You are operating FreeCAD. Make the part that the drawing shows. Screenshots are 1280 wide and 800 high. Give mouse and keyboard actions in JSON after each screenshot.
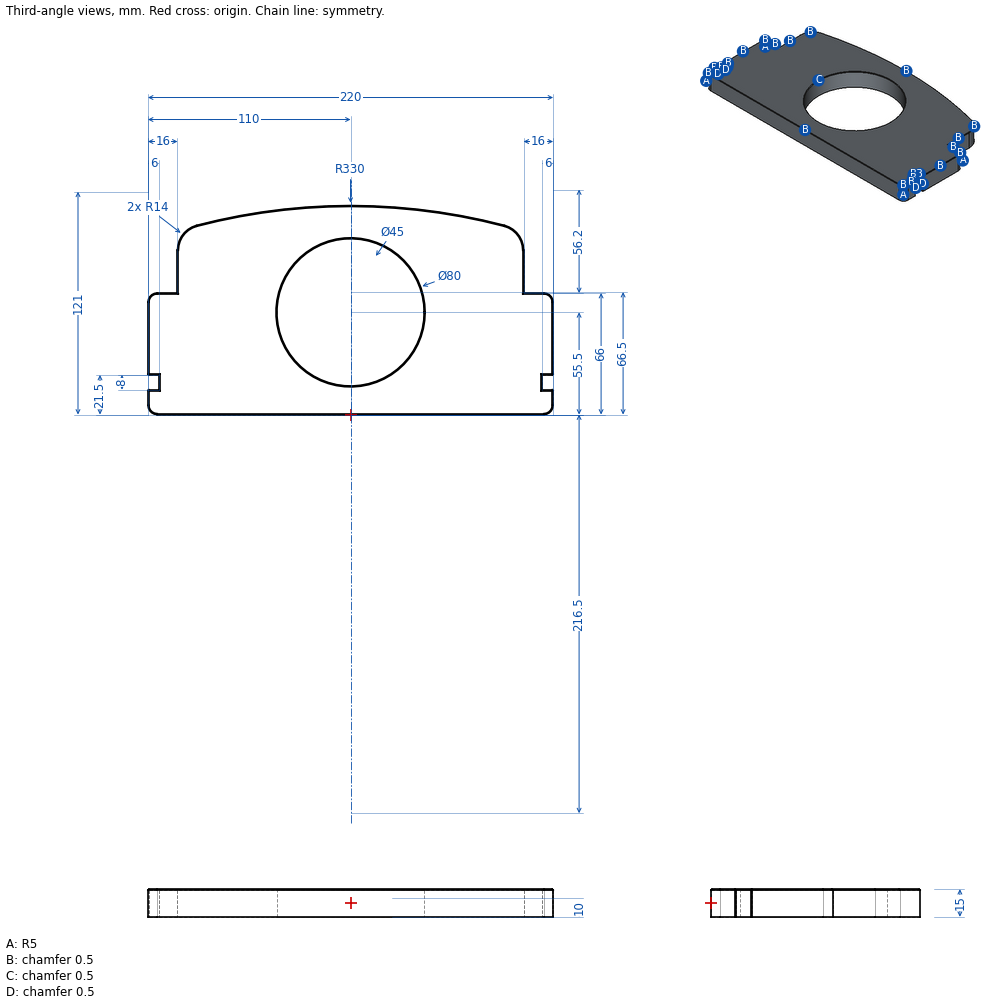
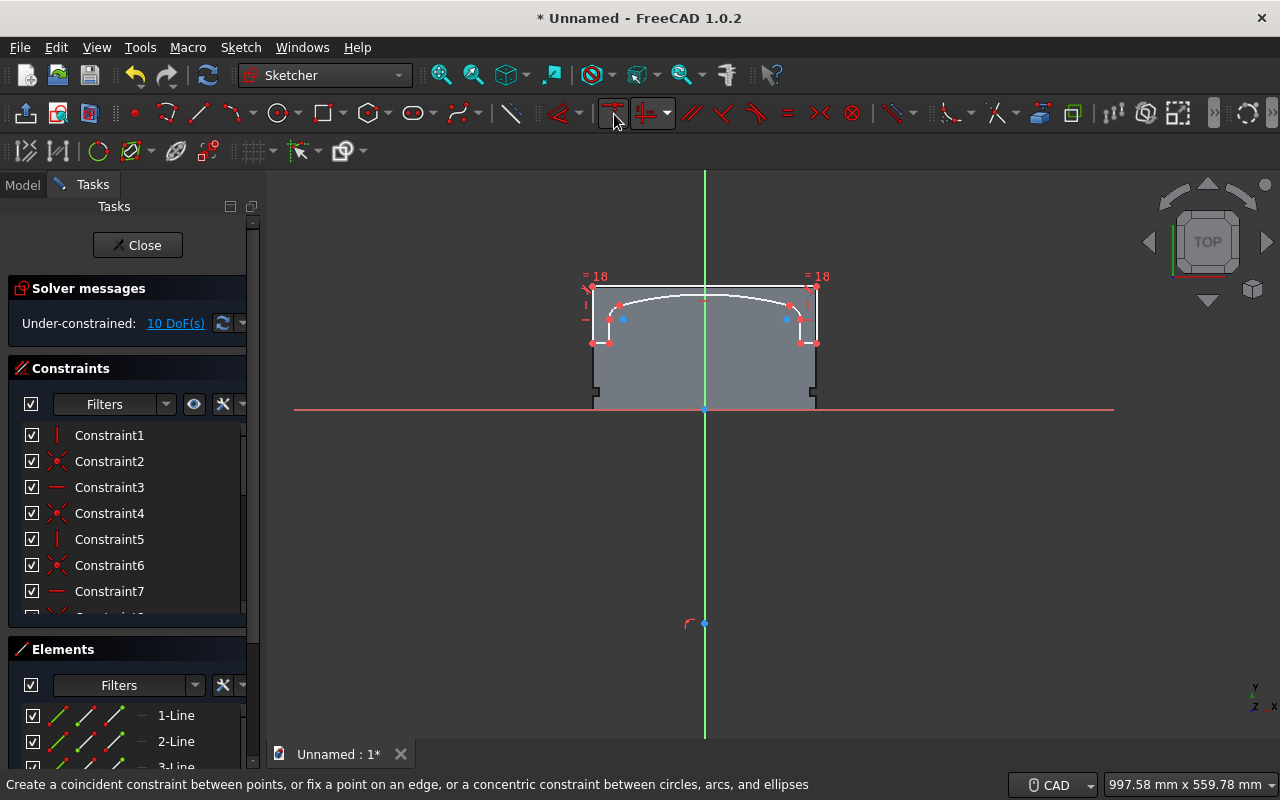
{"action": "left_click", "coordinate": [817, 343]}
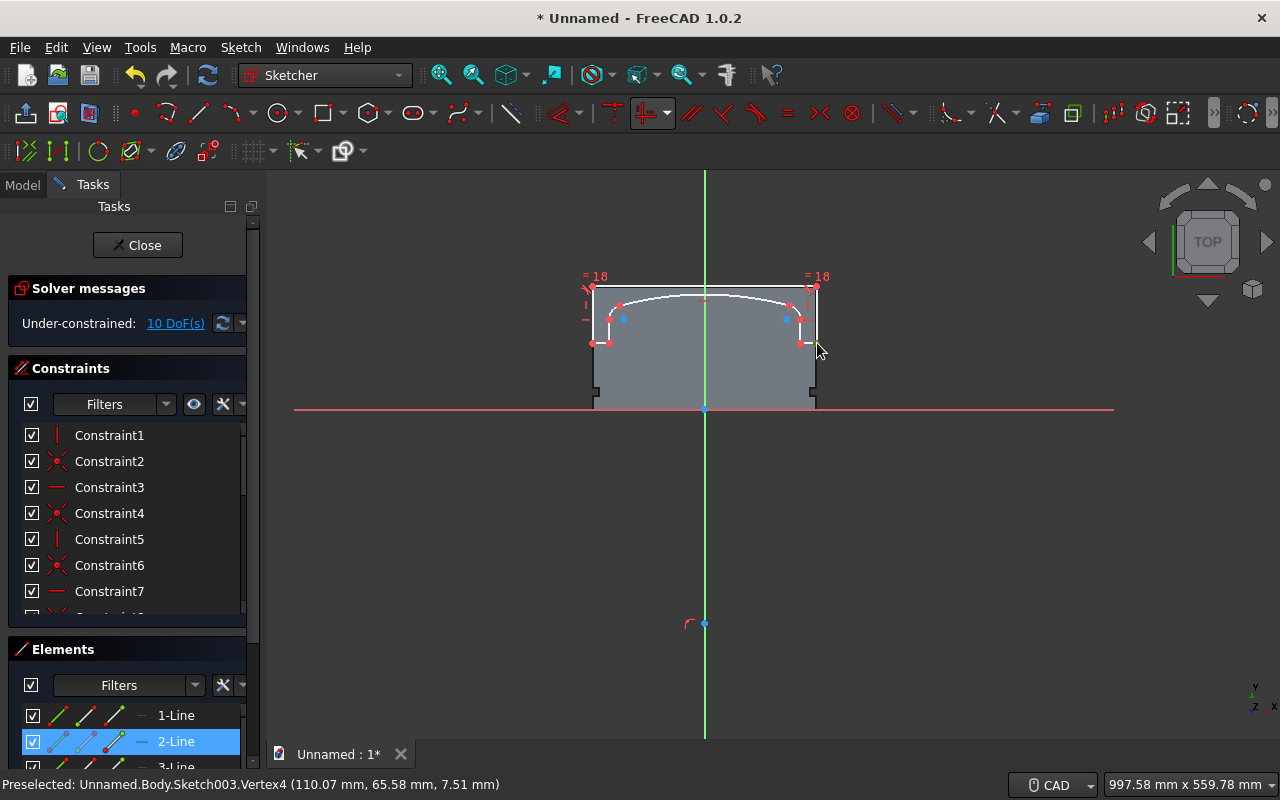
{"action": "left_click", "coordinate": [593, 343]}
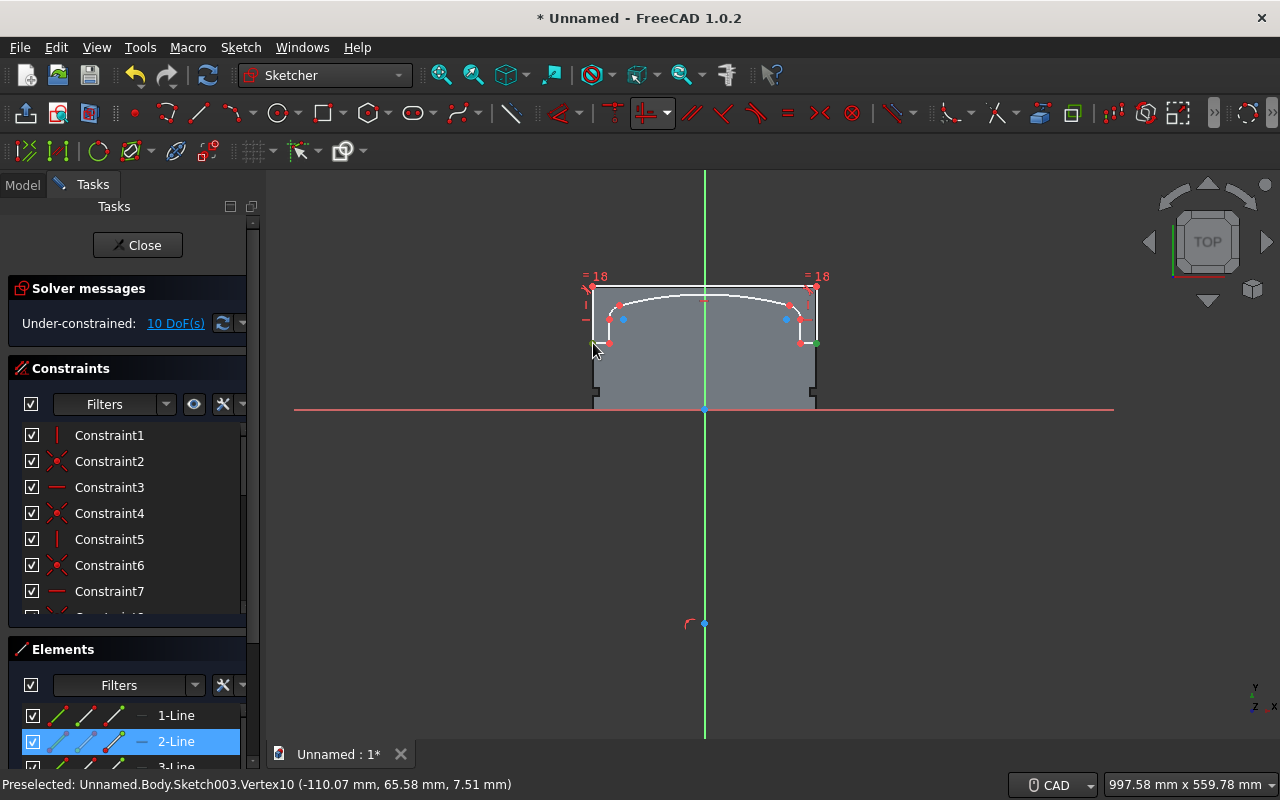
{"action": "left_click", "coordinate": [705, 674]}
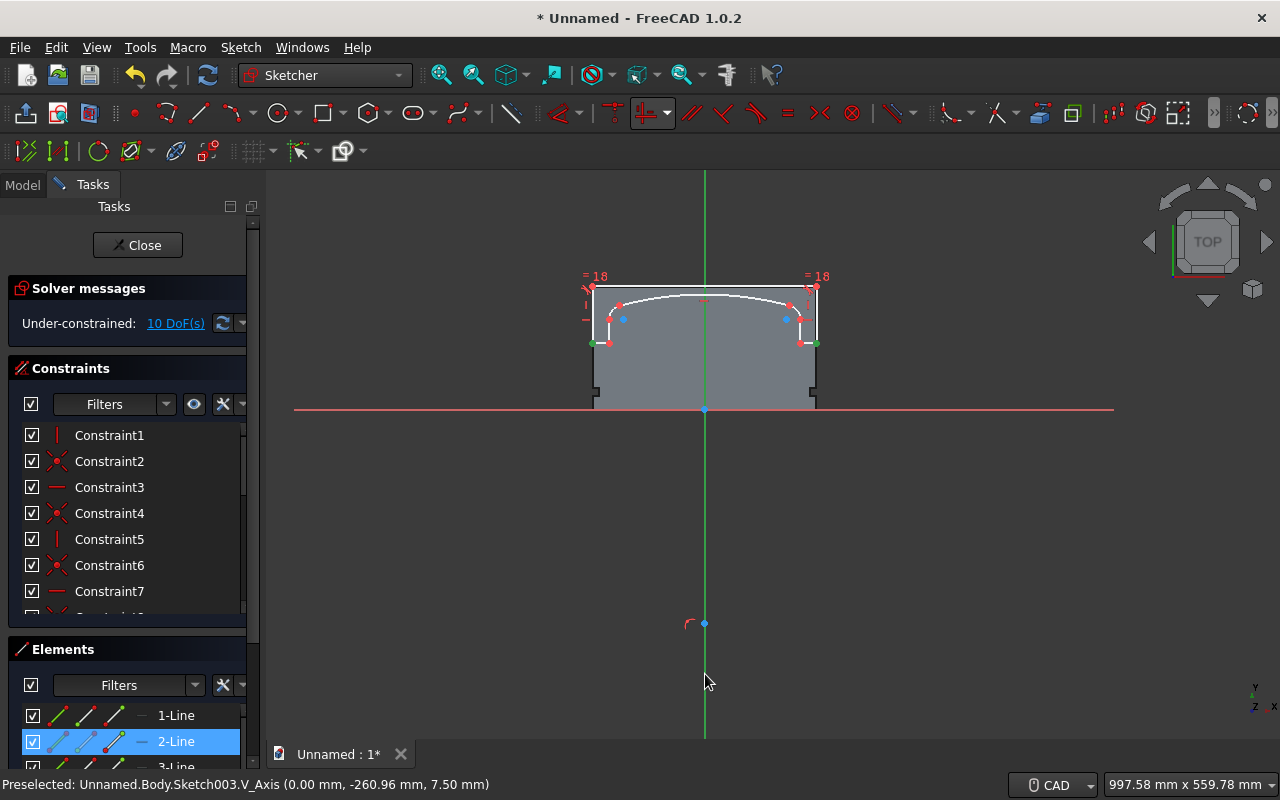
{"action": "left_click", "coordinate": [820, 114]}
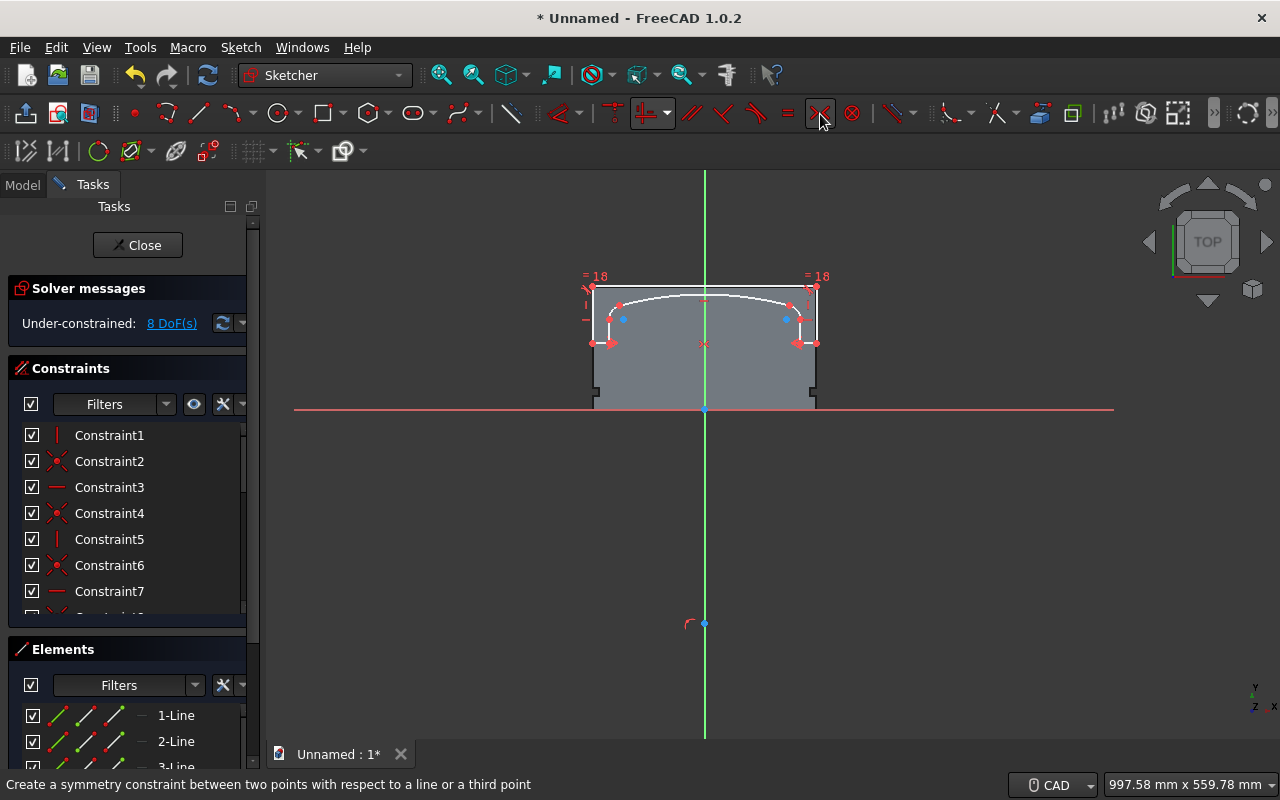
{"action": "left_click", "coordinate": [558, 114]}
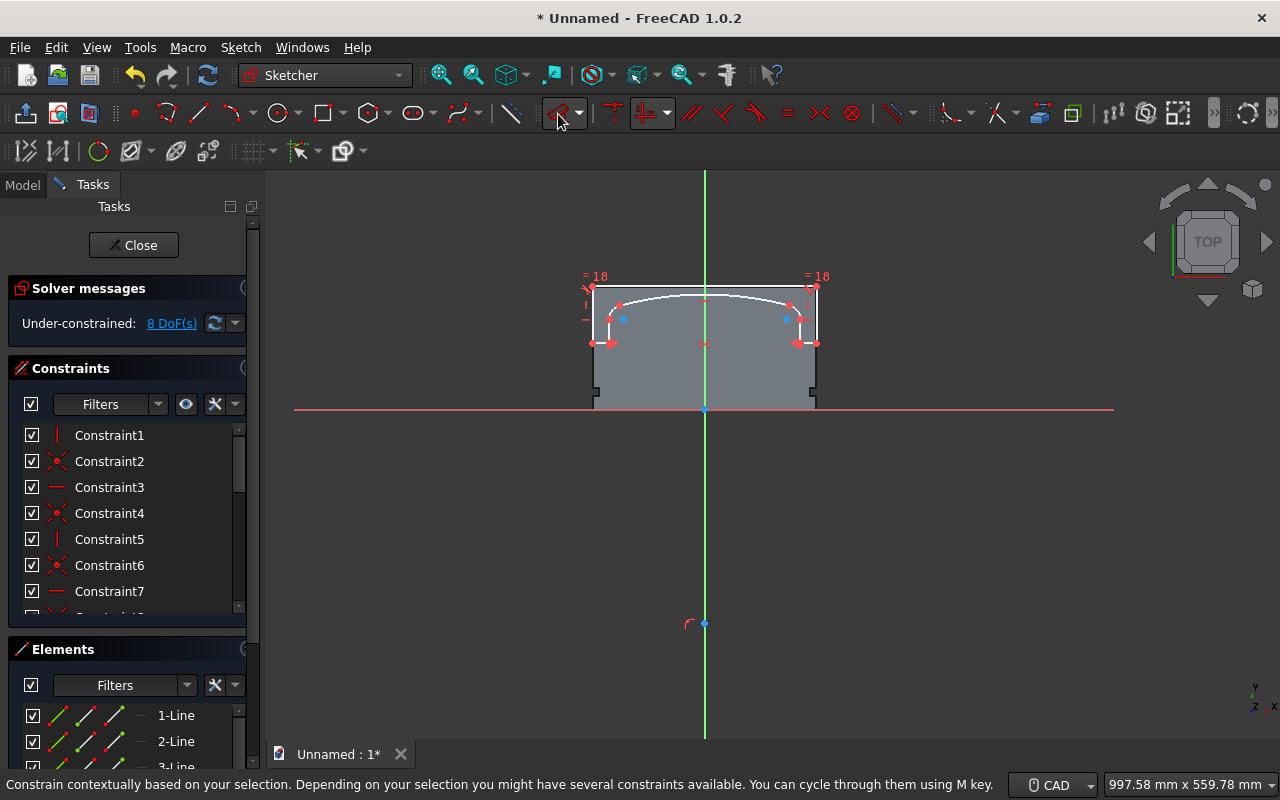
{"action": "scroll", "coordinate": [612, 311], "scroll_direction": "up", "scroll_amount": 6}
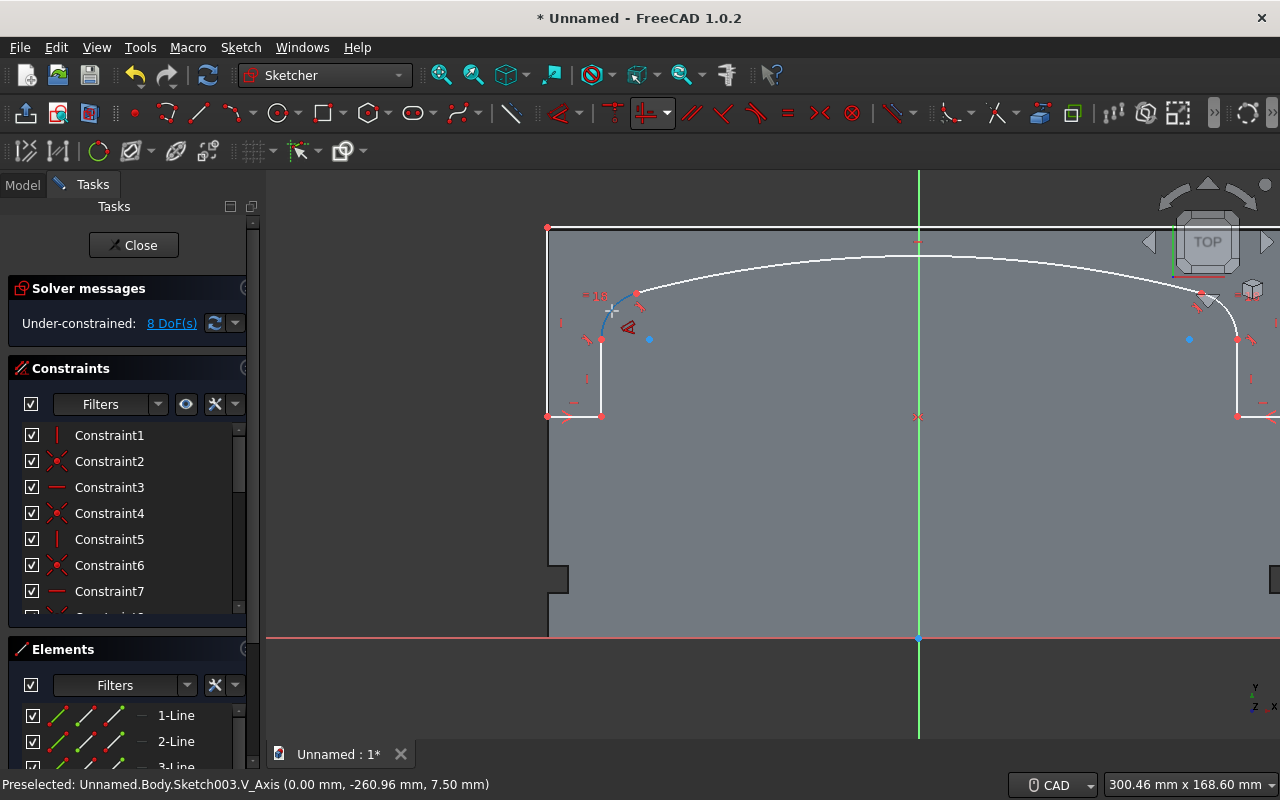
{"action": "left_click", "coordinate": [611, 310]}
{"action": "left_click", "coordinate": [586, 291]}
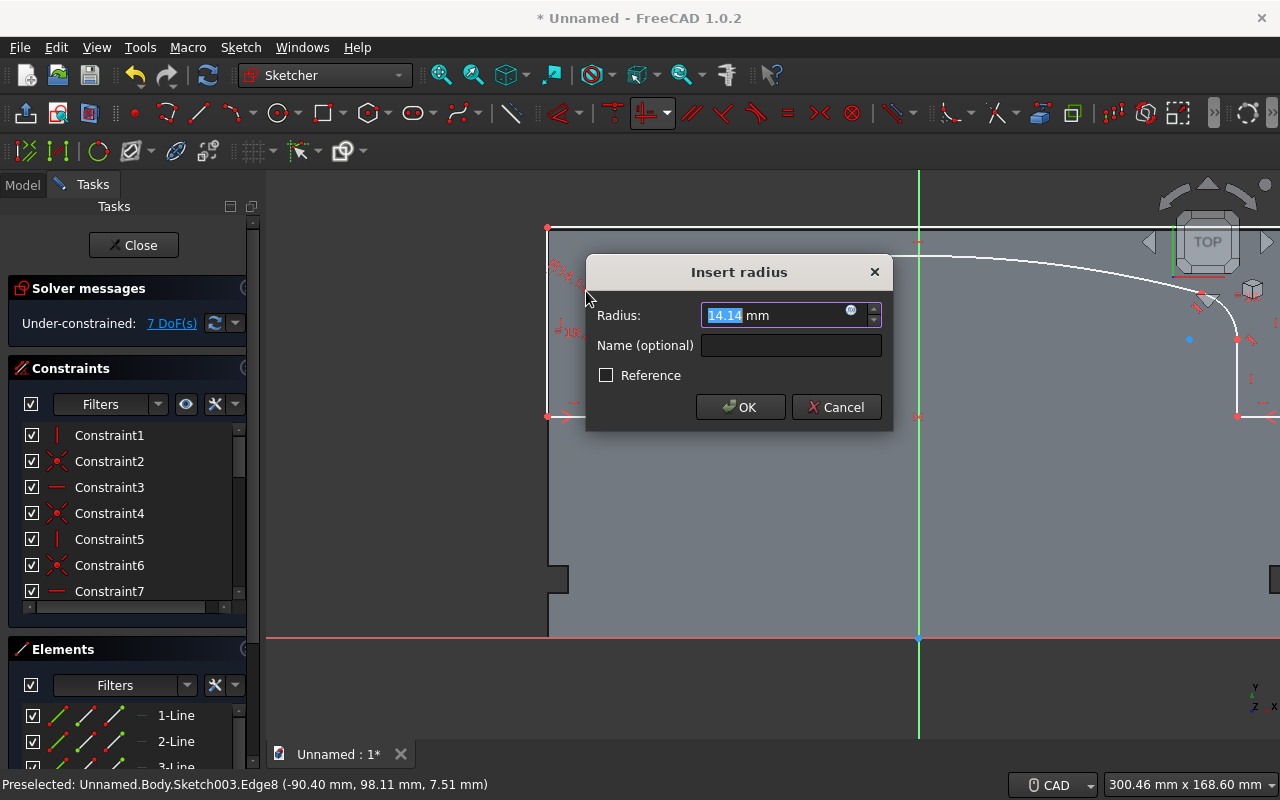
{"action": "type", "text": "14"}
{"action": "key", "text": "Return"}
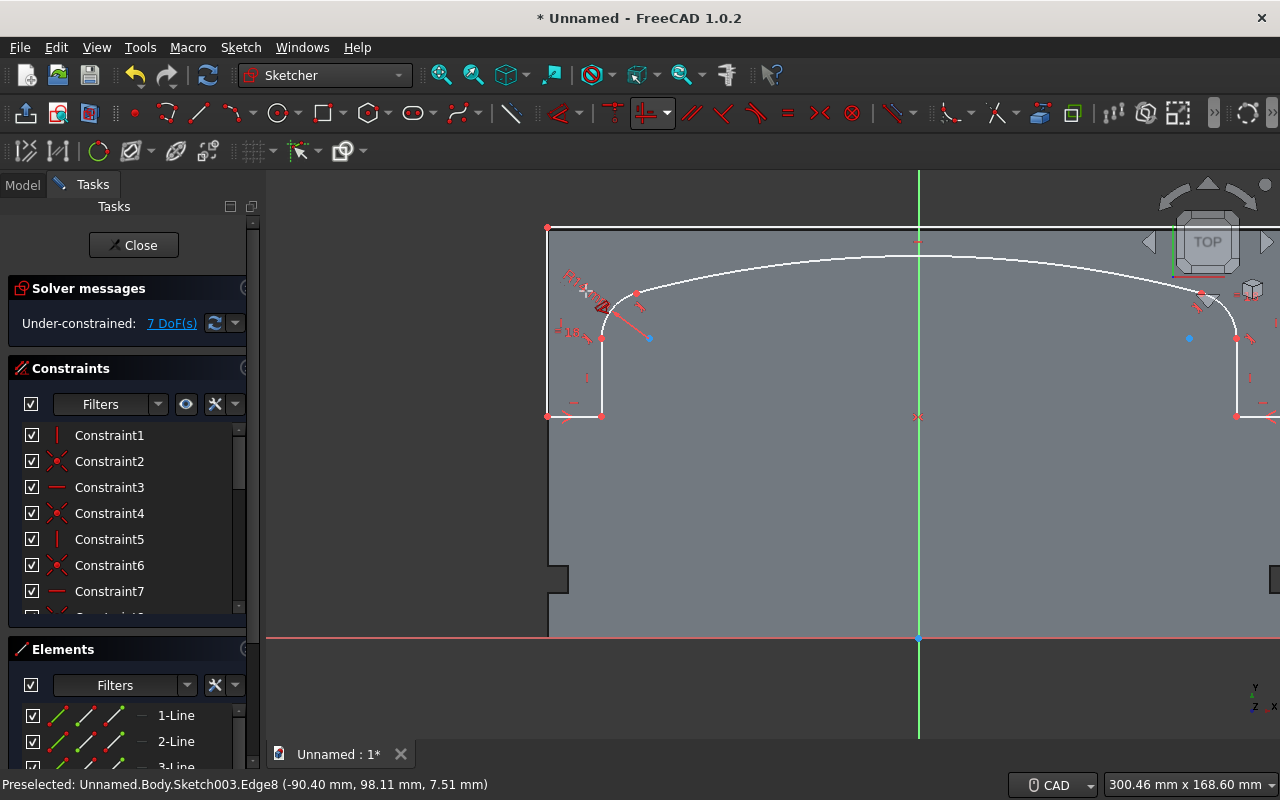
{"action": "left_click", "coordinate": [1033, 262]}
{"action": "left_click", "coordinate": [486, 311]}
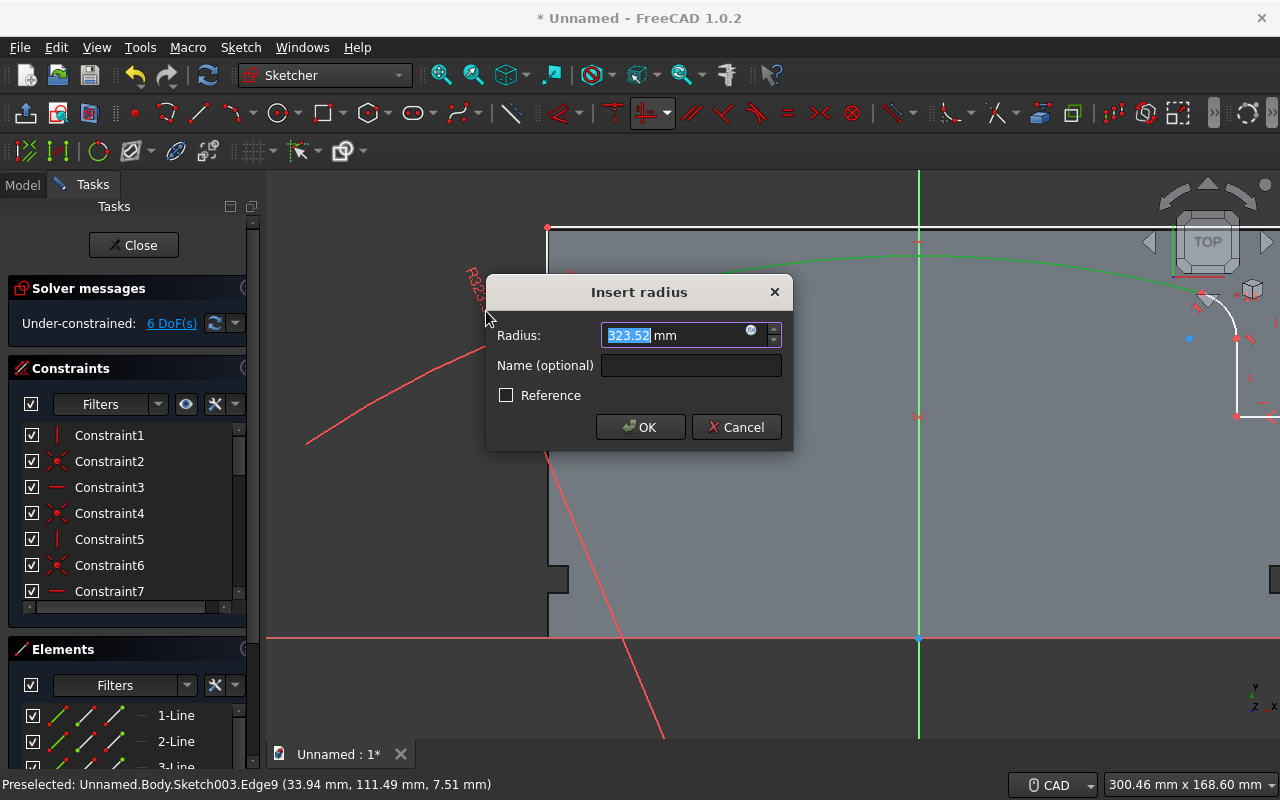
{"action": "type", "text": "330"}
{"action": "key", "text": "Return"}